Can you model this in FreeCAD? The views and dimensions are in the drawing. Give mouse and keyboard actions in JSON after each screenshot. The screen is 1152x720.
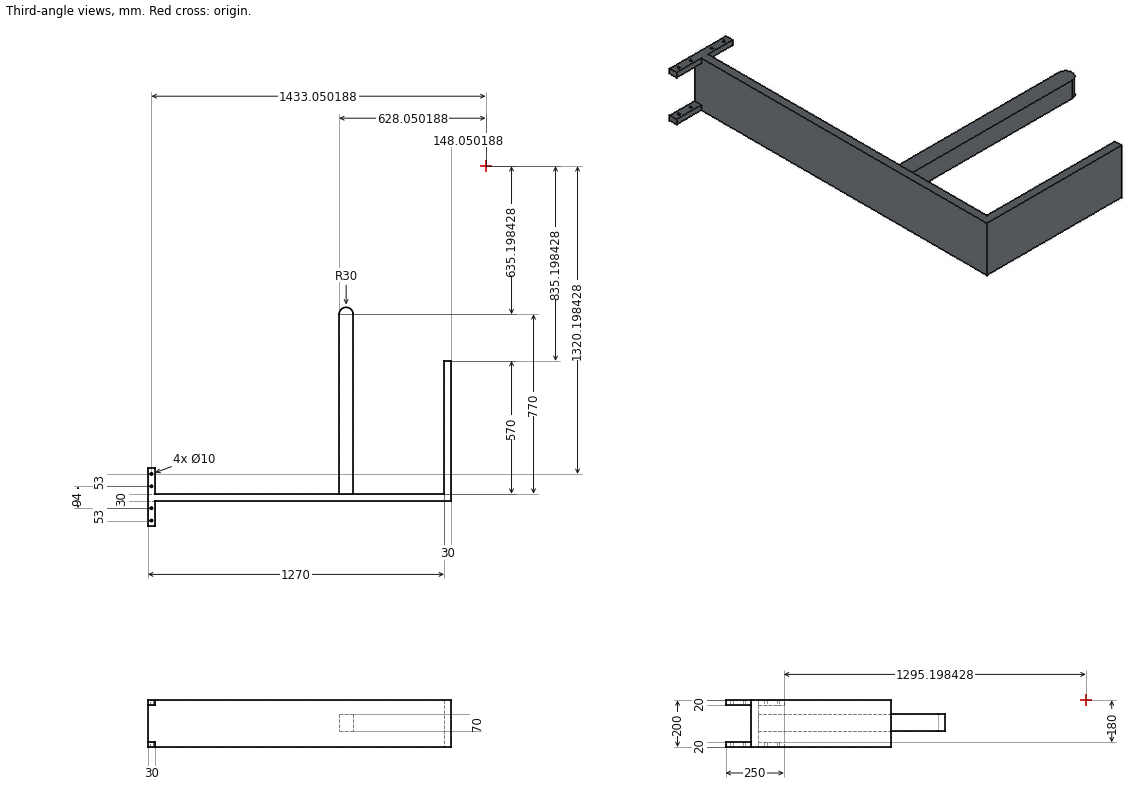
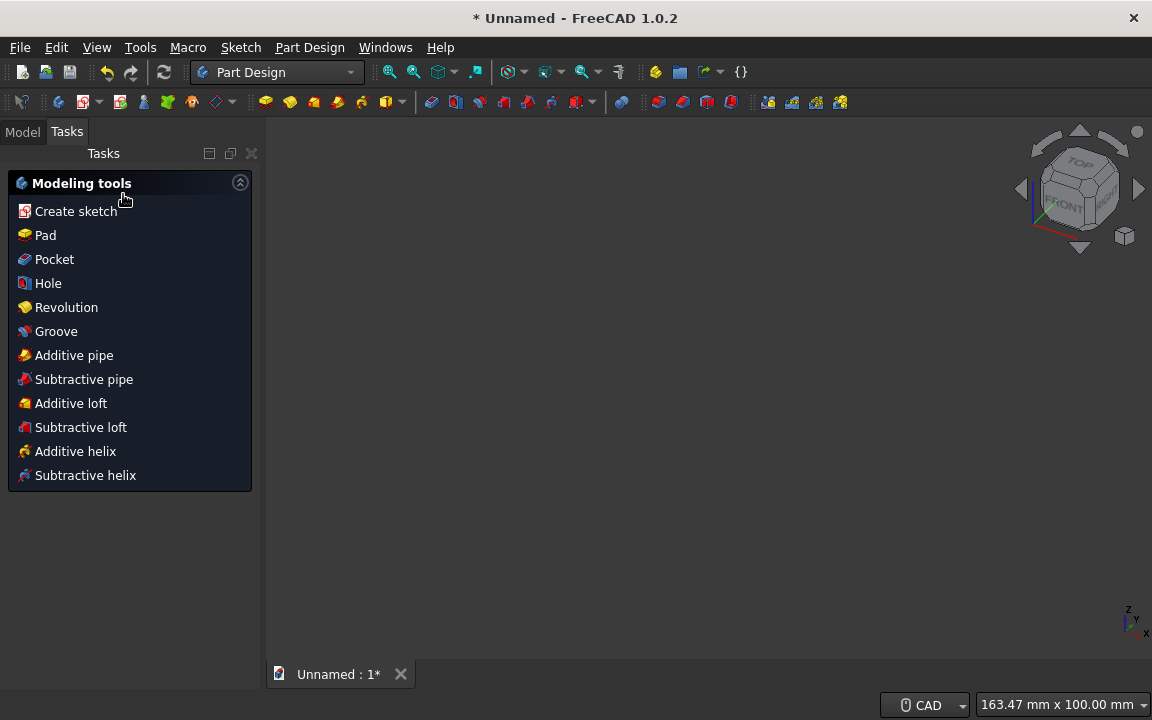
{"action": "left_click", "coordinate": [266, 102]}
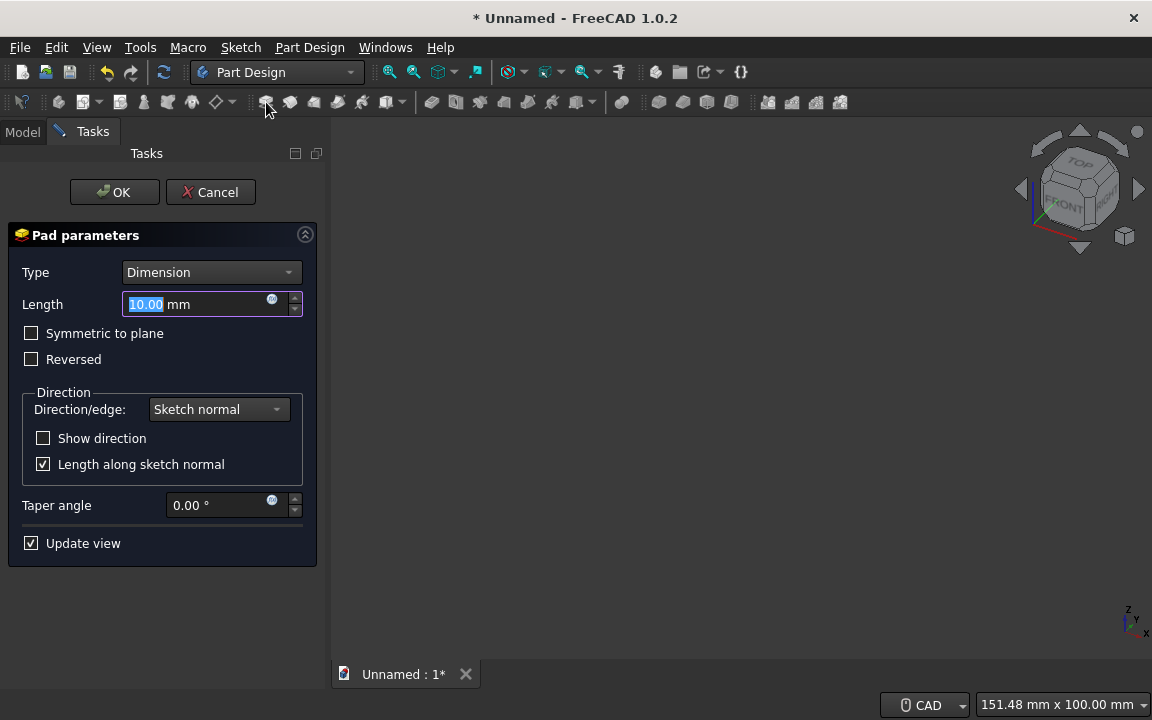
{"action": "type", "text": "200"}
{"action": "key", "text": "Tab"}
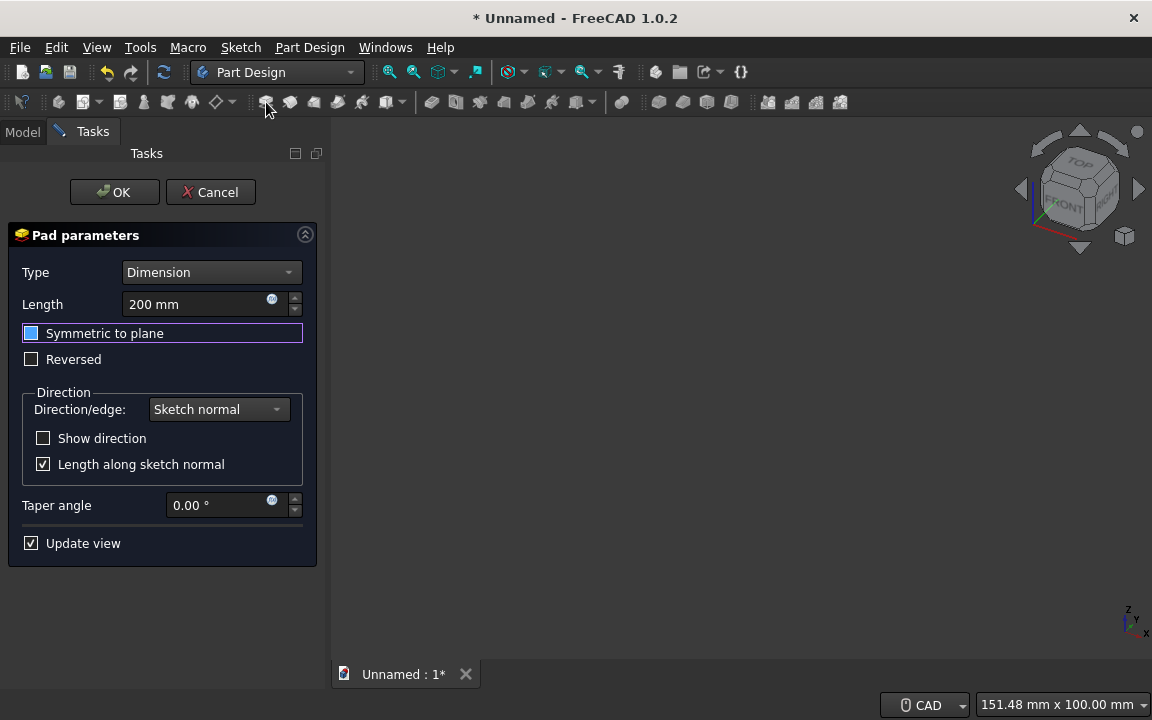
{"action": "left_click", "coordinate": [30, 359]}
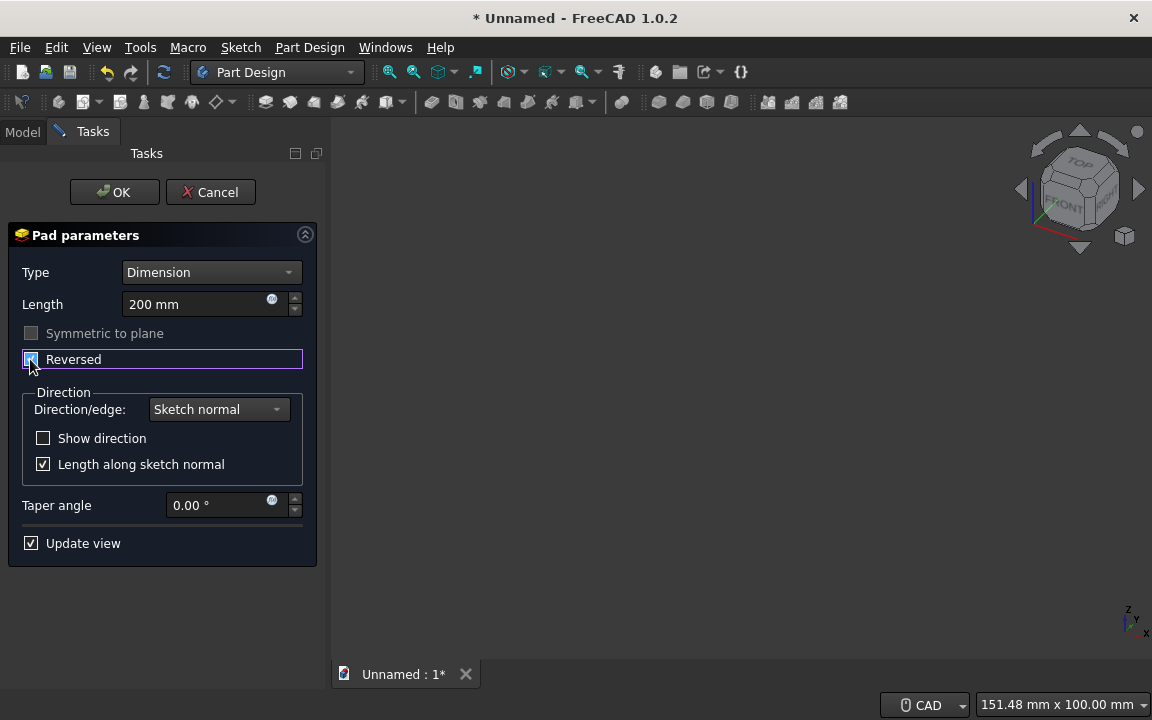
{"action": "left_click", "coordinate": [115, 192]}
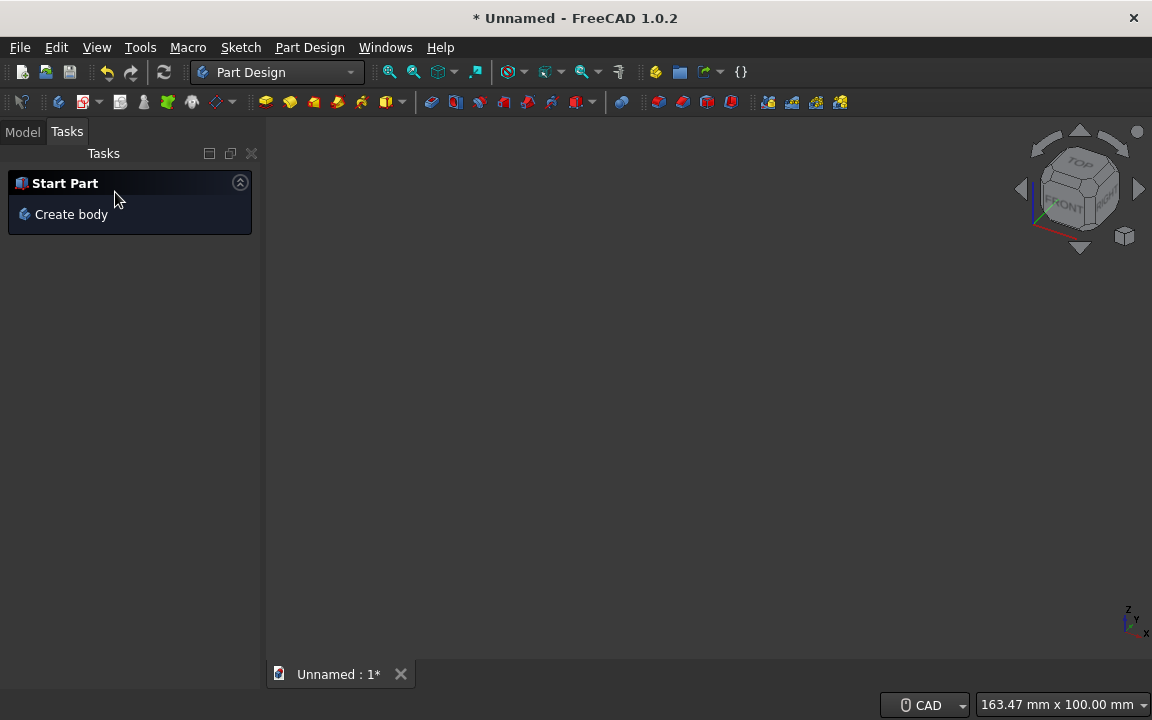
{"action": "left_click", "coordinate": [390, 72]}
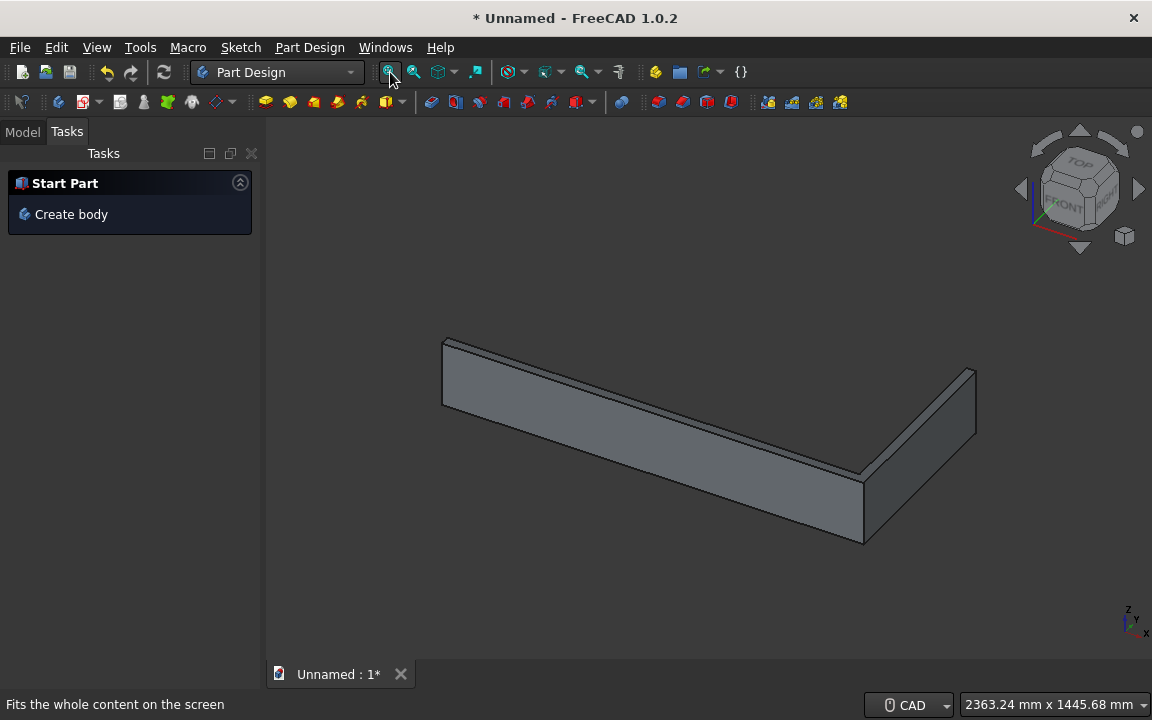
{"action": "key", "text": "6"}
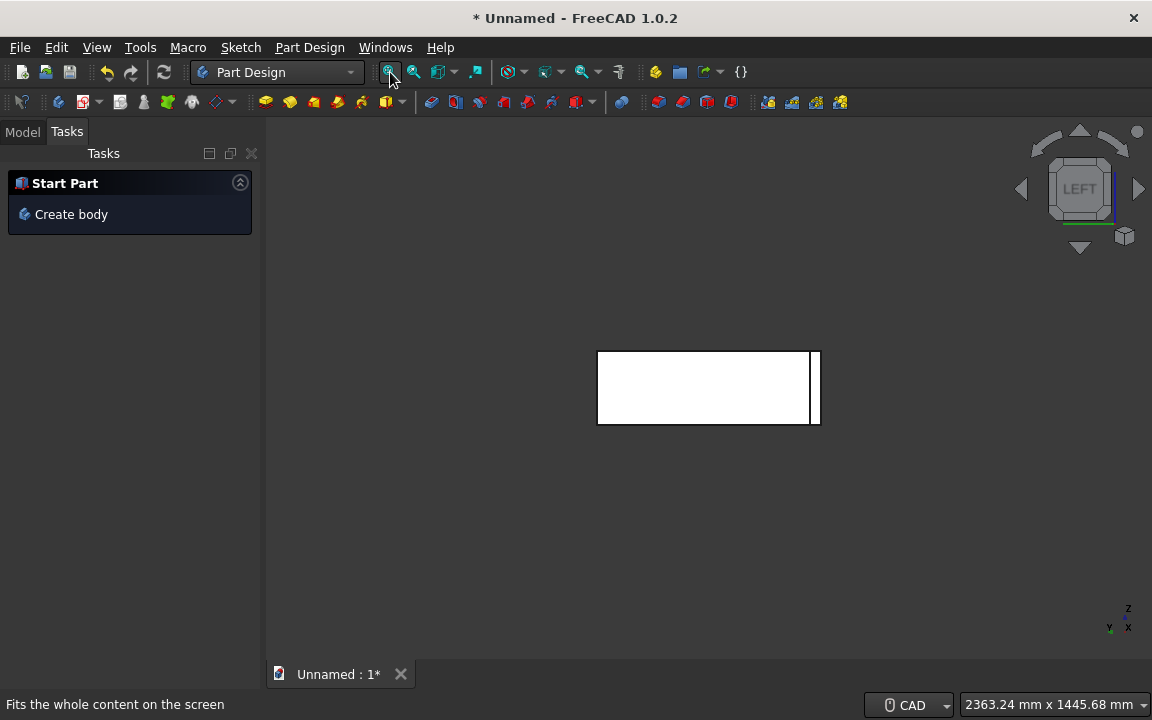
{"action": "left_click", "coordinate": [390, 72]}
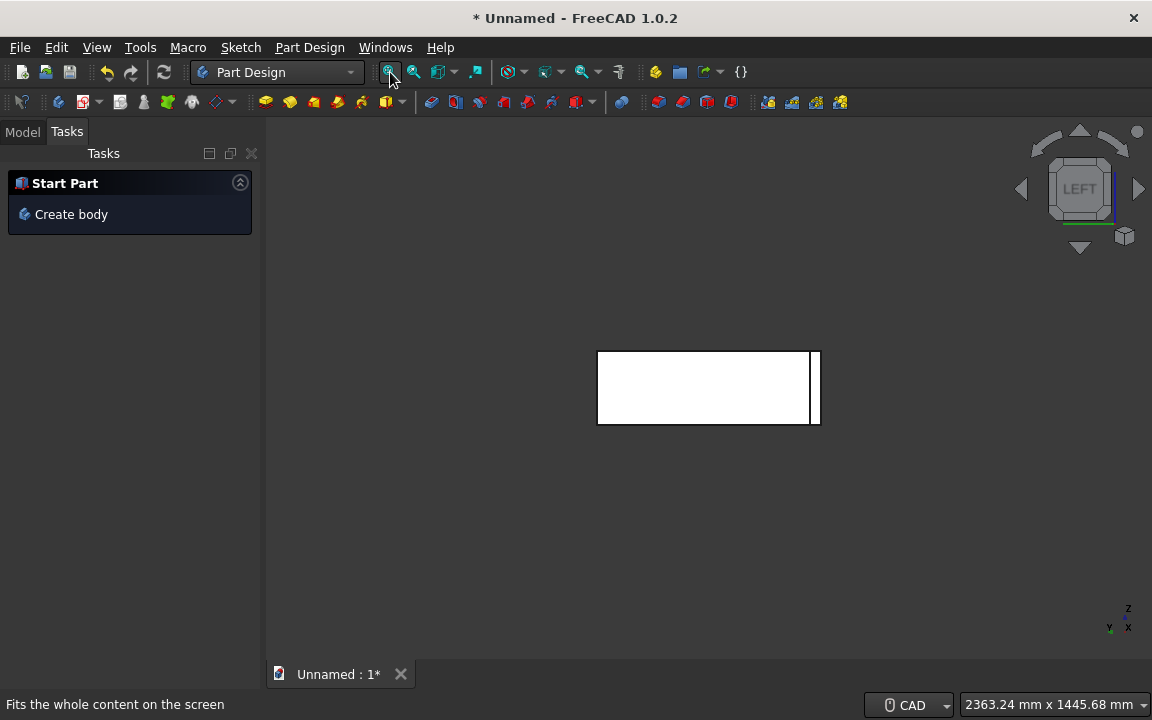
{"action": "scroll", "coordinate": [816, 366], "scroll_direction": "up", "scroll_amount": 4}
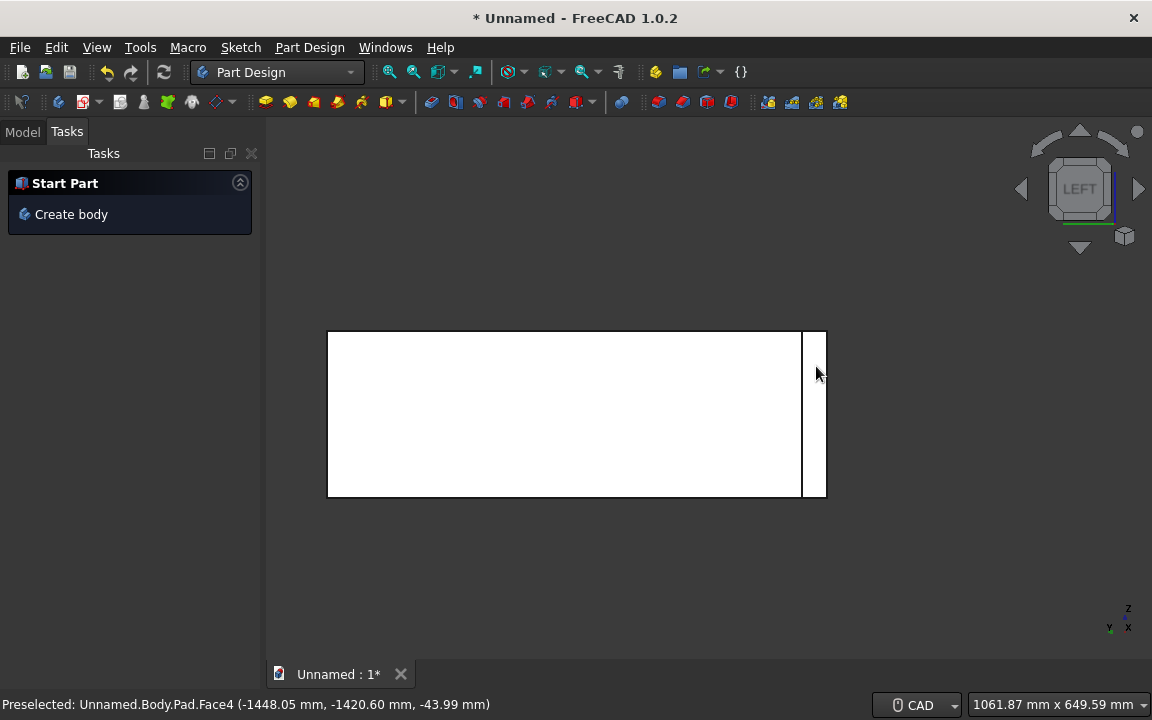
{"action": "left_click", "coordinate": [815, 366]}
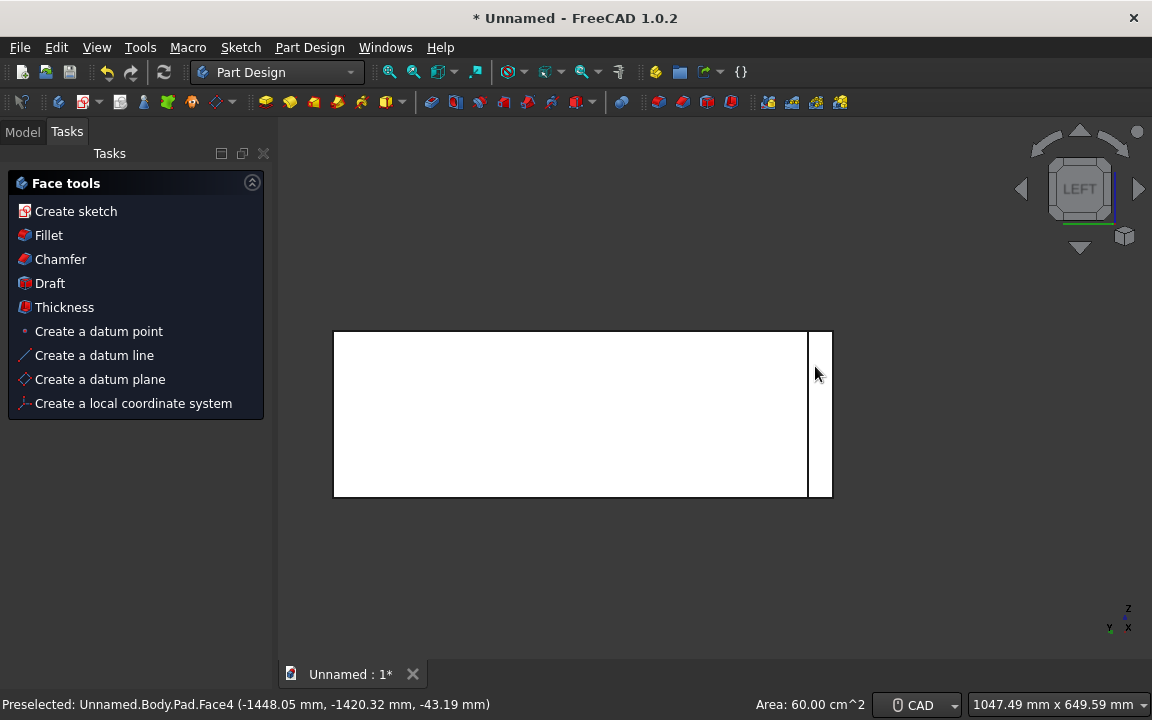
{"action": "left_click", "coordinate": [84, 102]}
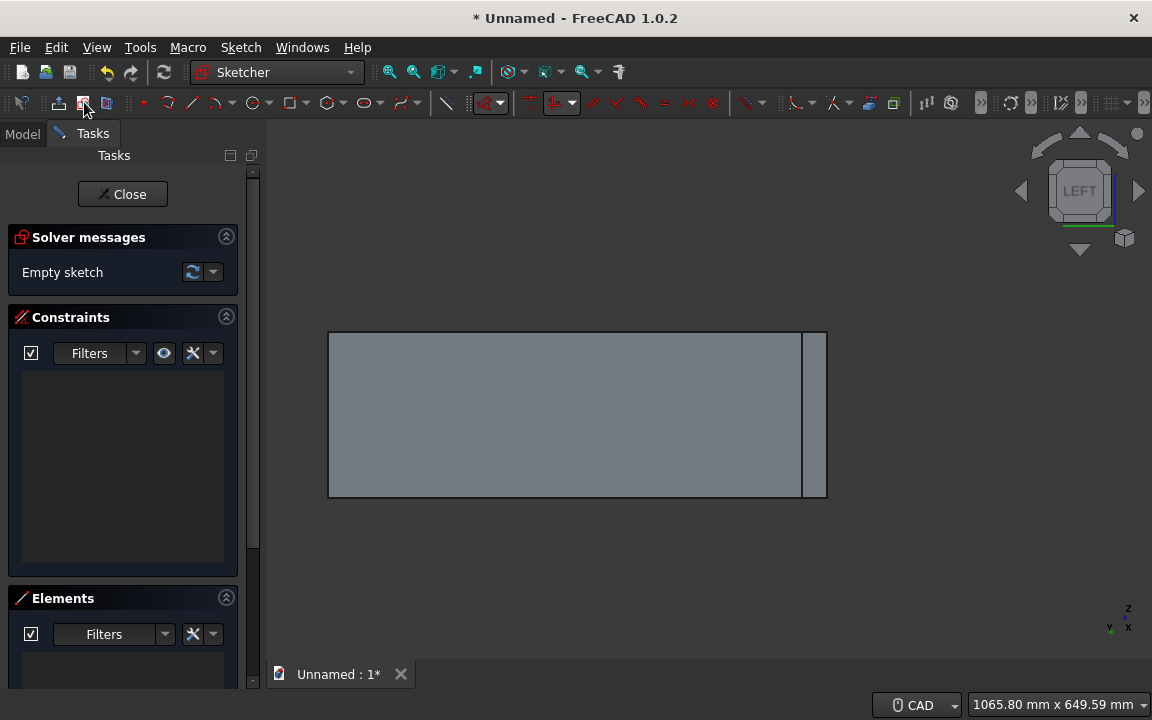
{"action": "scroll", "coordinate": [956, 437], "scroll_direction": "up", "scroll_amount": 4}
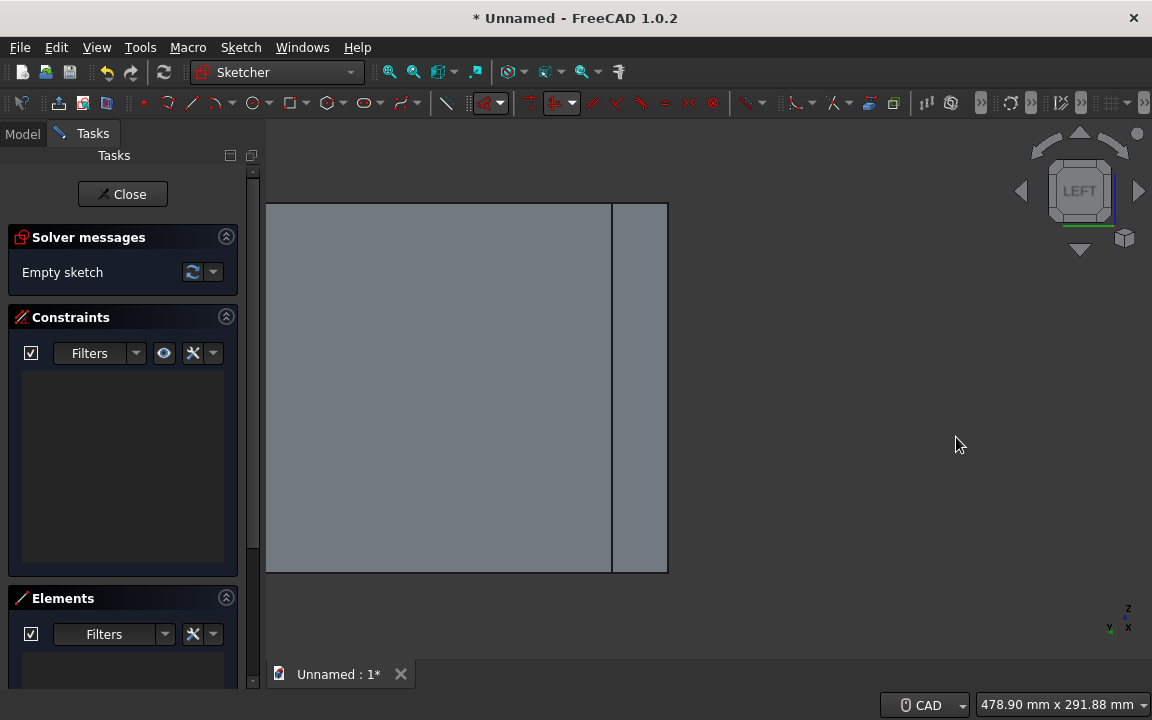
{"action": "left_click", "coordinate": [290, 104]}